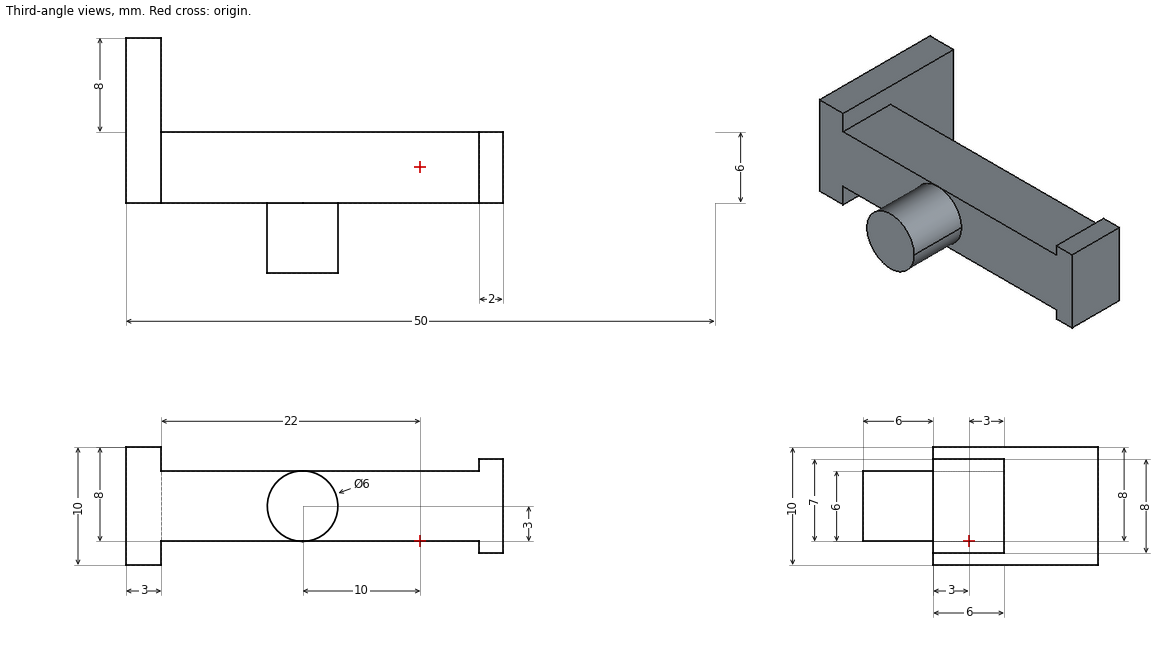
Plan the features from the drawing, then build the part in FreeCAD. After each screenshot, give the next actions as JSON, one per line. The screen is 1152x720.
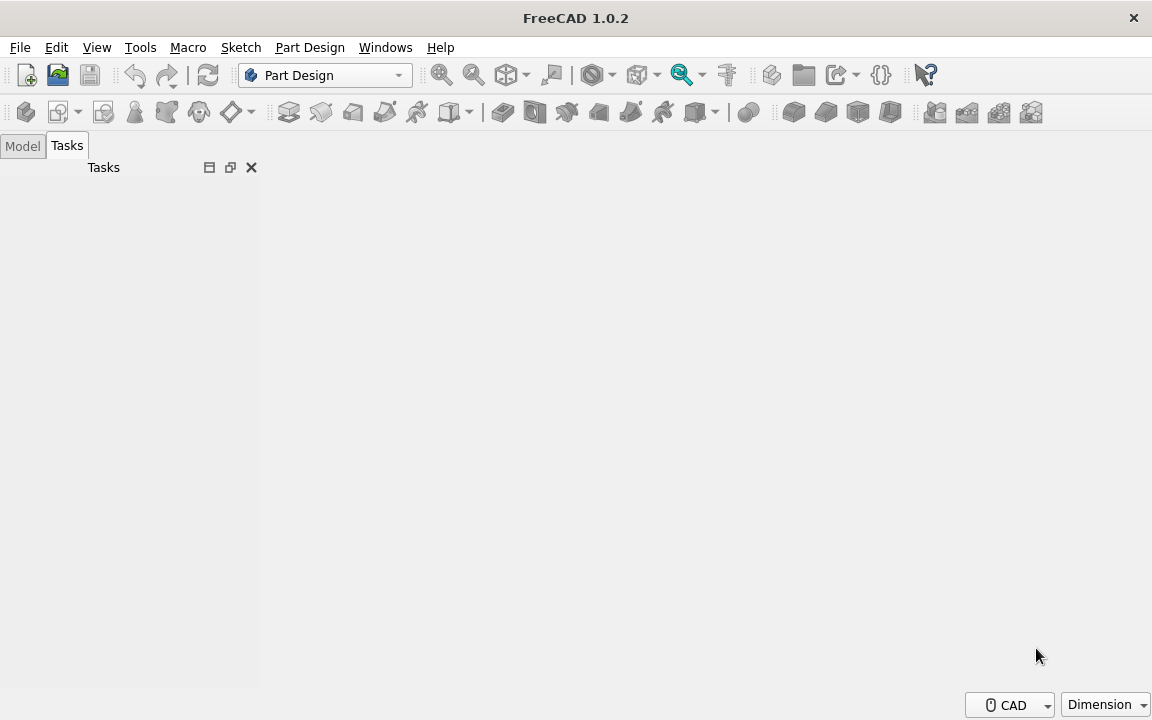
{"action": "left_click", "coordinate": [26, 76]}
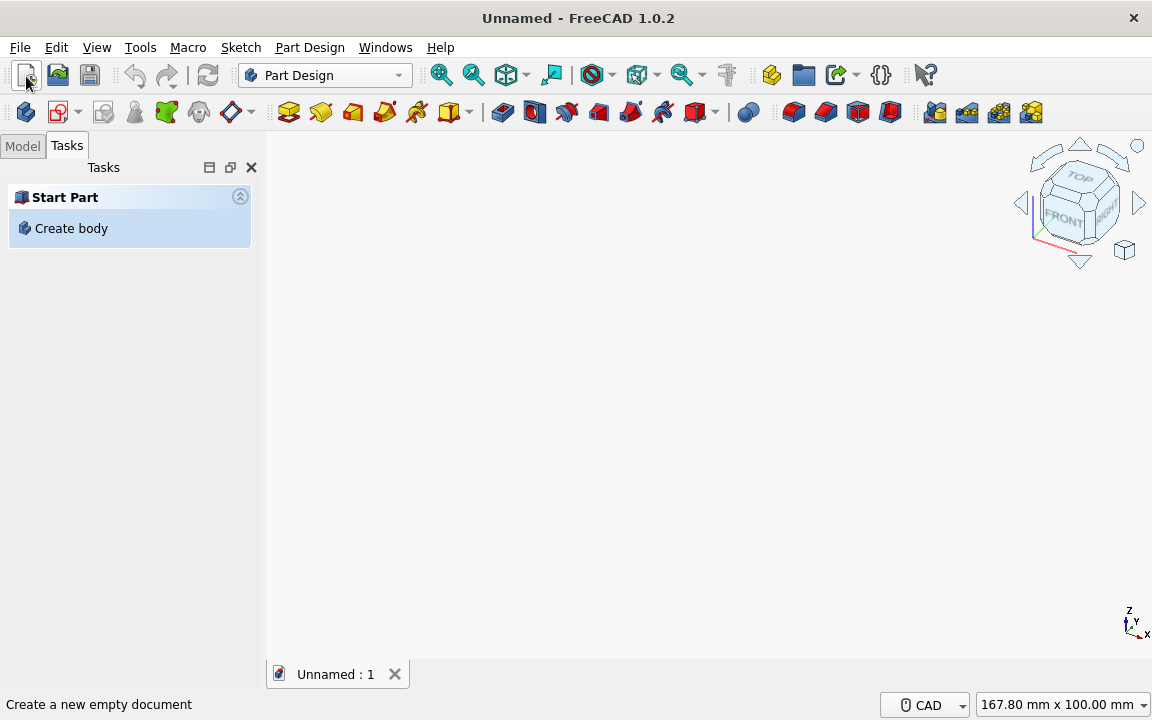
{"action": "left_click", "coordinate": [58, 112]}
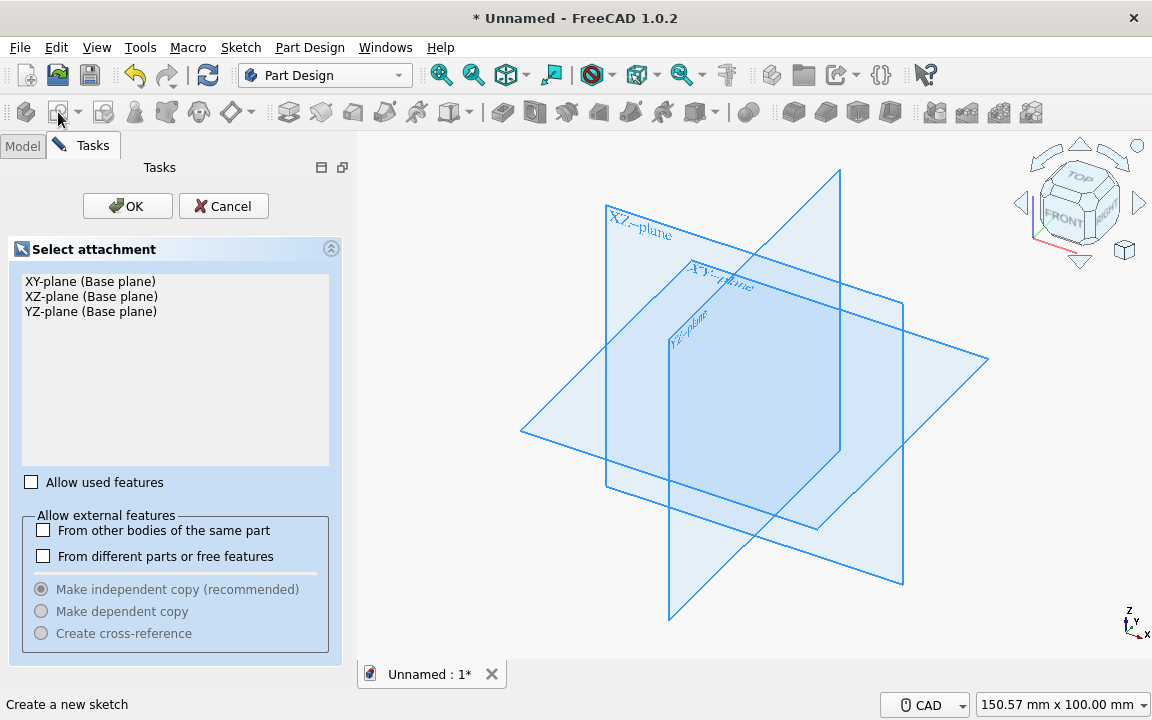
{"action": "left_click", "coordinate": [82, 282]}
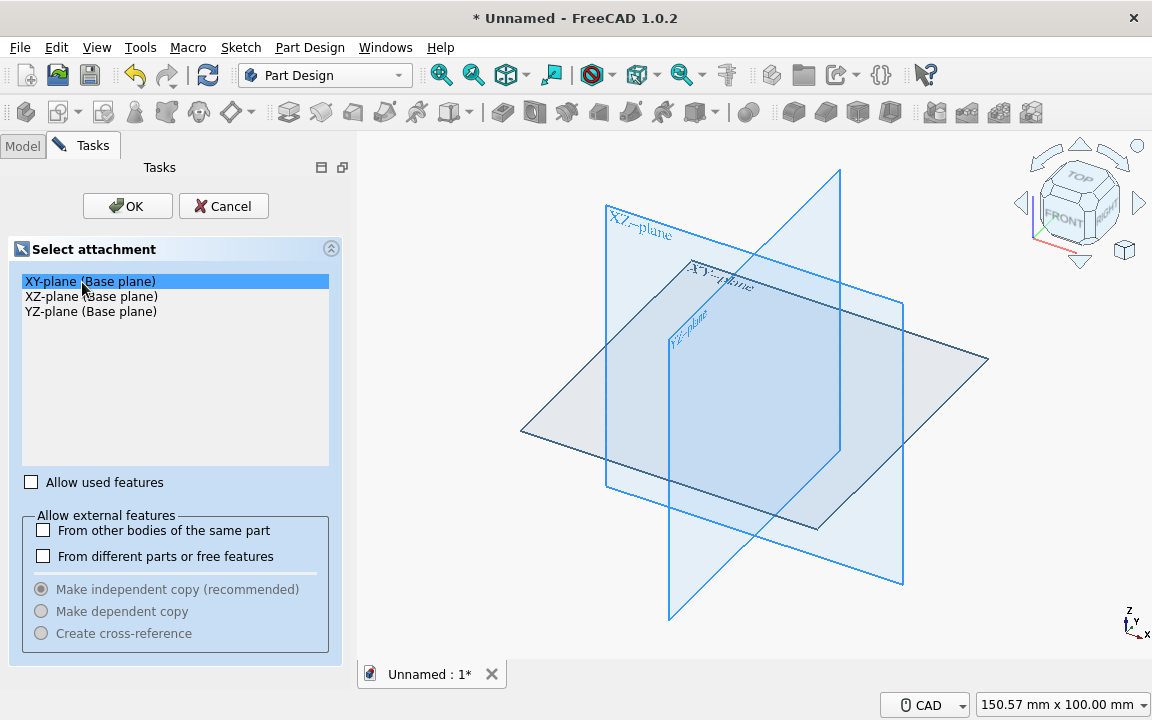
{"action": "left_click", "coordinate": [128, 206]}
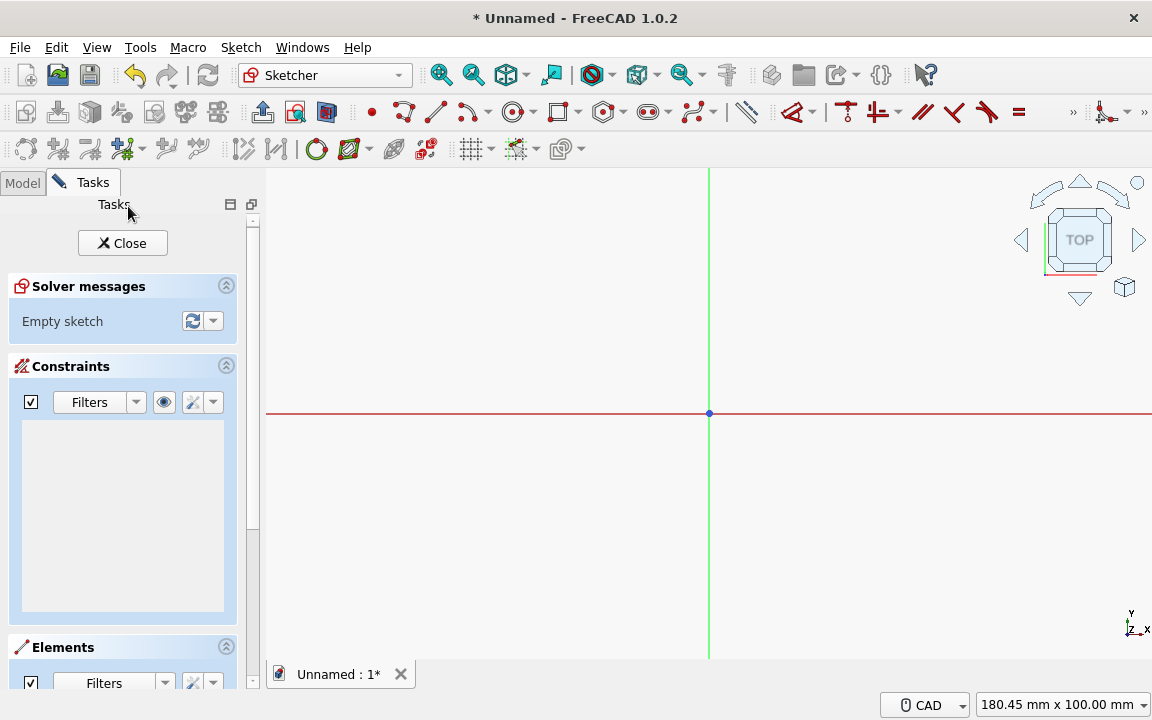
{"action": "scroll", "coordinate": [792, 414], "scroll_direction": "up", "scroll_amount": 3}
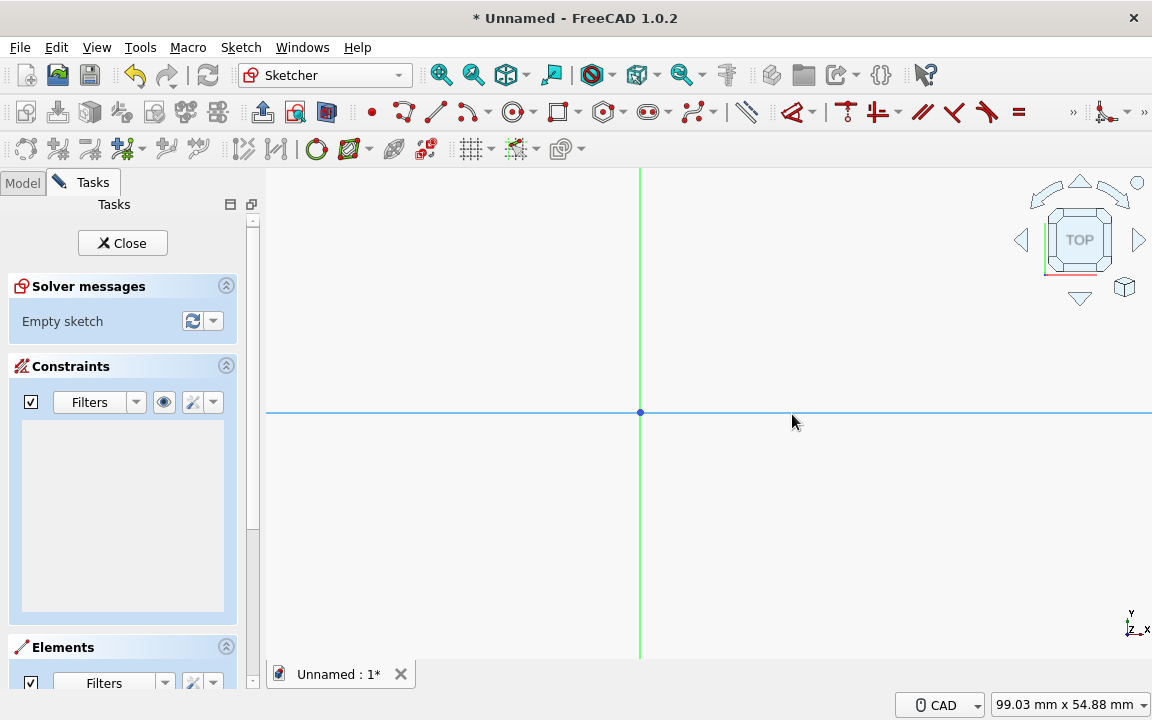
{"action": "key", "text": "g v"}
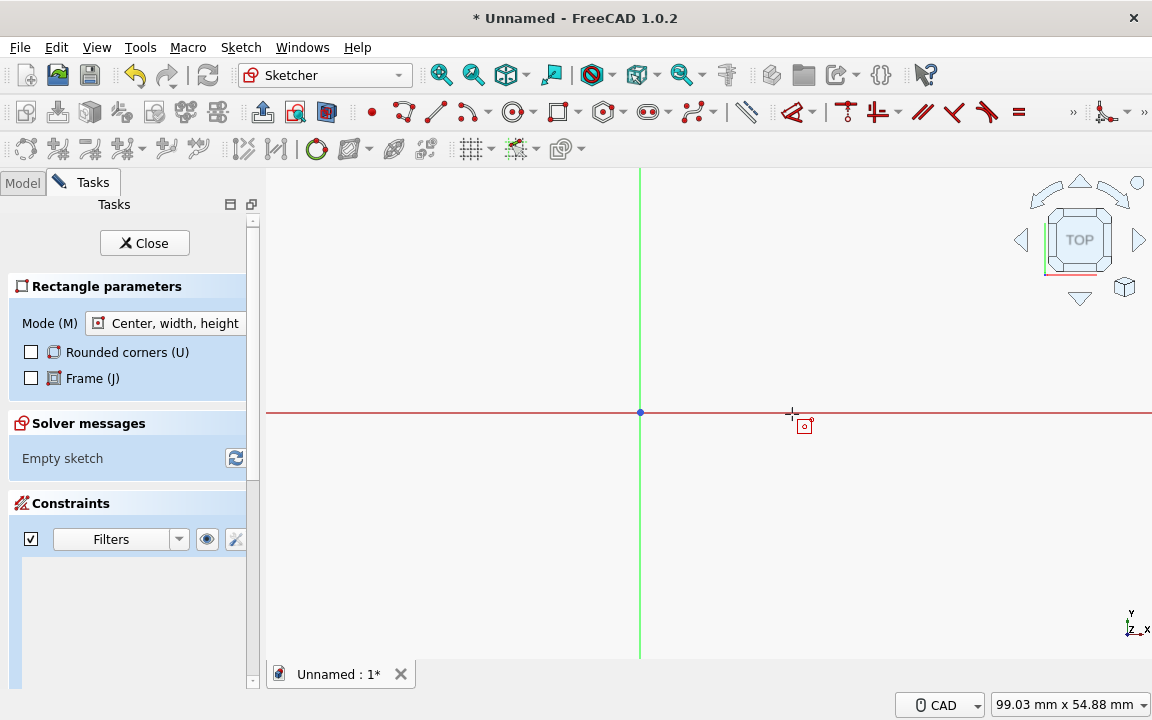
{"action": "left_click", "coordinate": [640, 413]}
{"action": "mouse_move", "coordinate": [864, 386]}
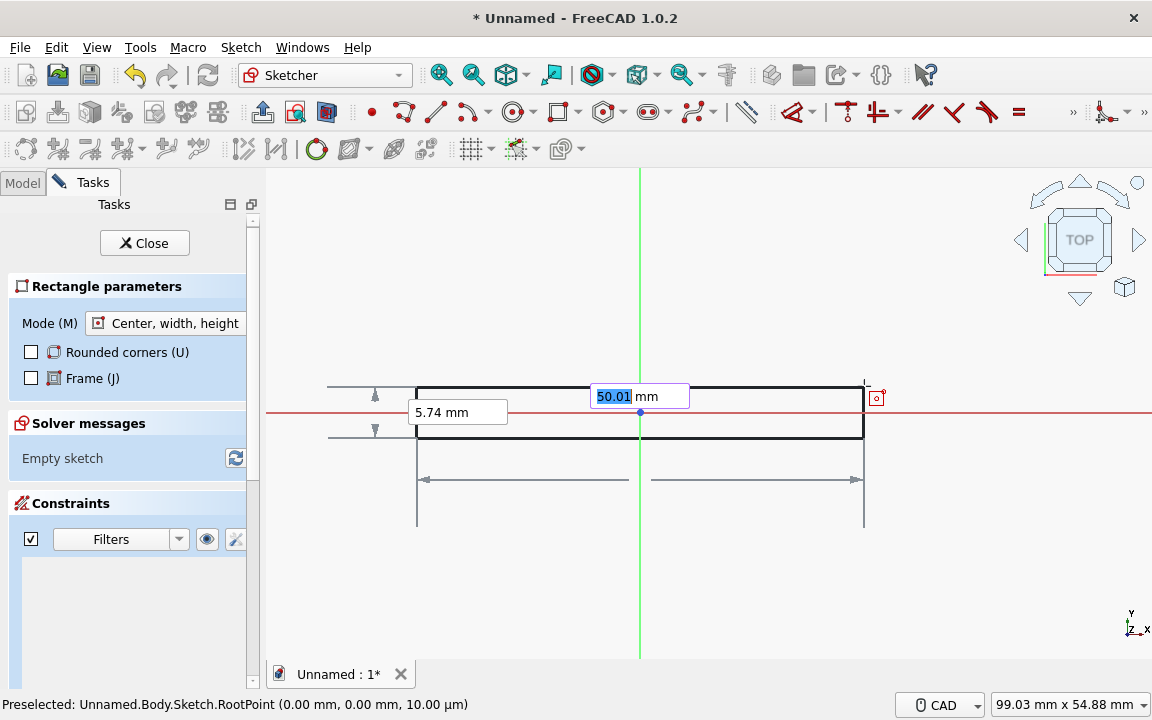
{"action": "type", "text": "50"}
{"action": "key", "text": "Tab"}
{"action": "type", "text": "6"}
{"action": "key", "text": "Return"}
{"action": "key", "text": "Escape"}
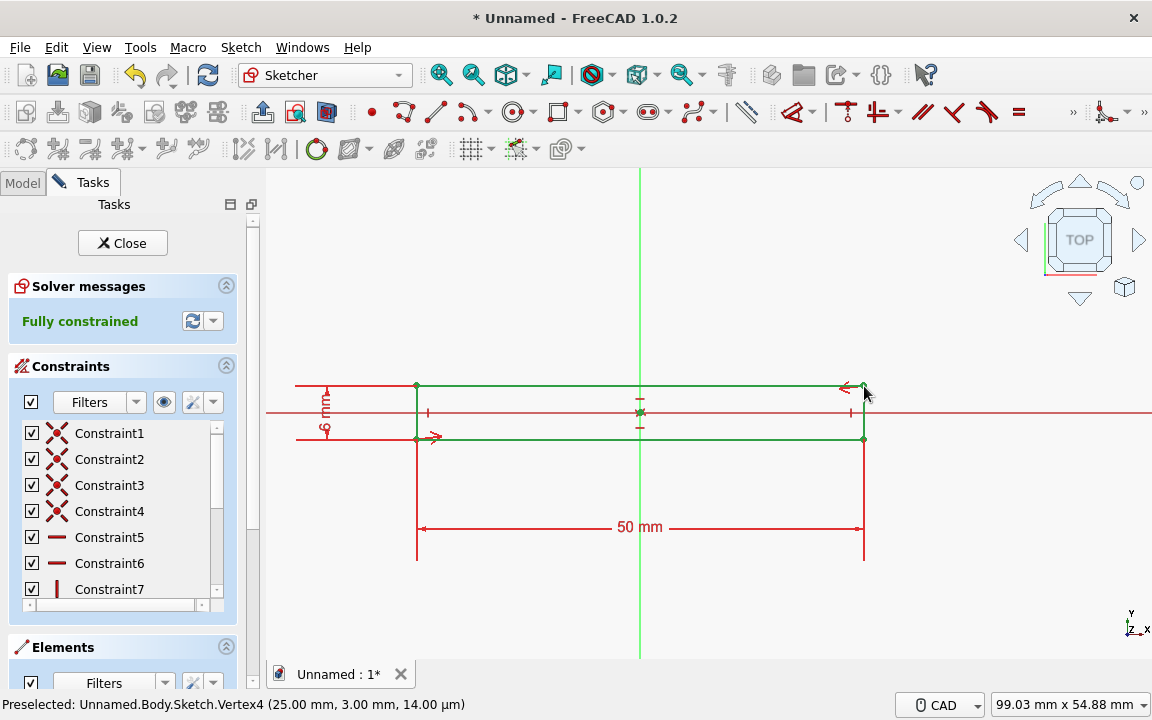
{"action": "left_click", "coordinate": [123, 243]}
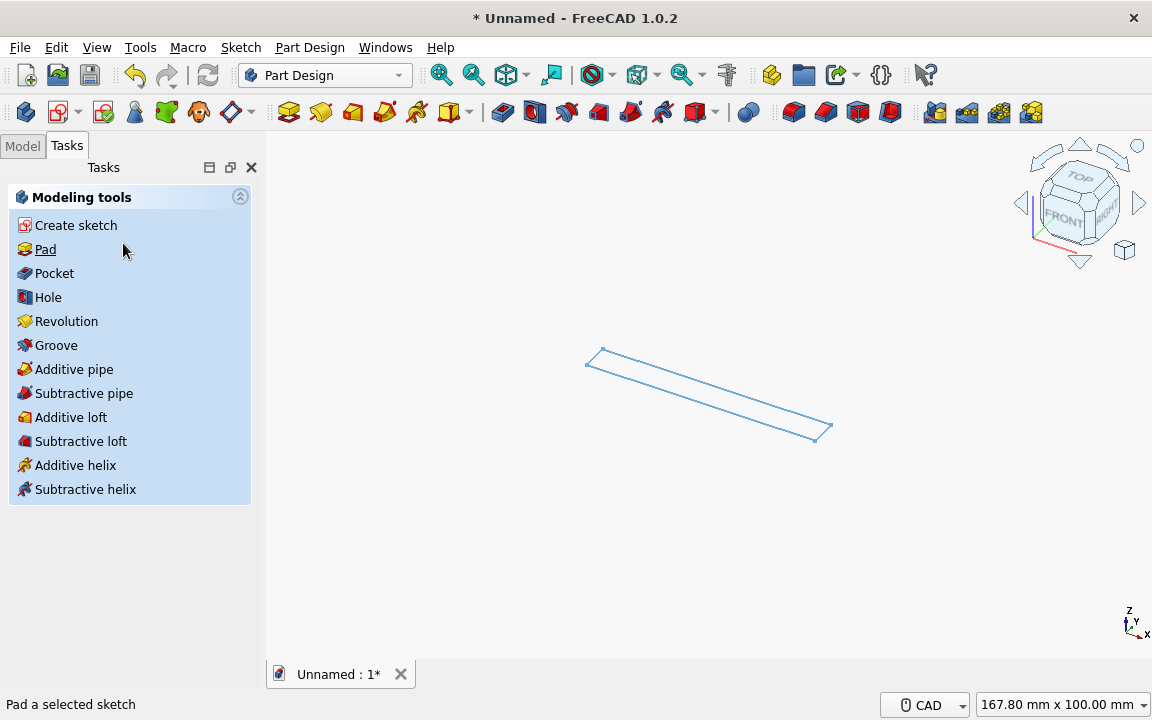
{"action": "left_click", "coordinate": [290, 112]}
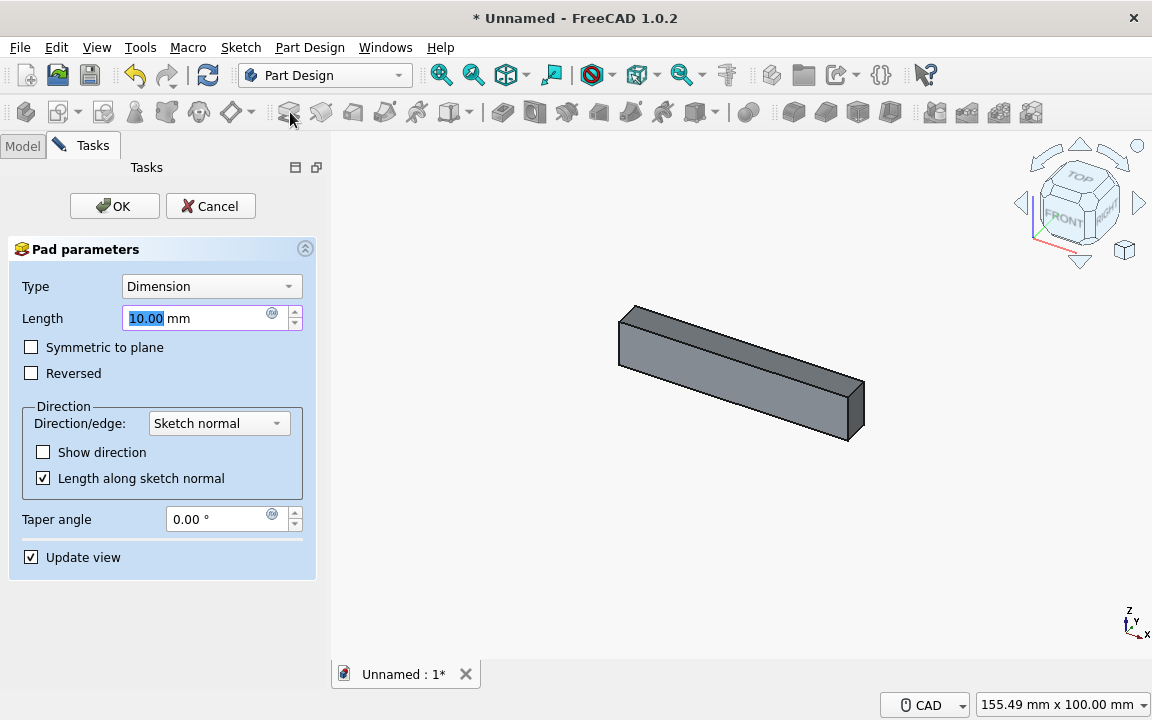
{"action": "type", "text": "6"}
{"action": "key", "text": "Tab"}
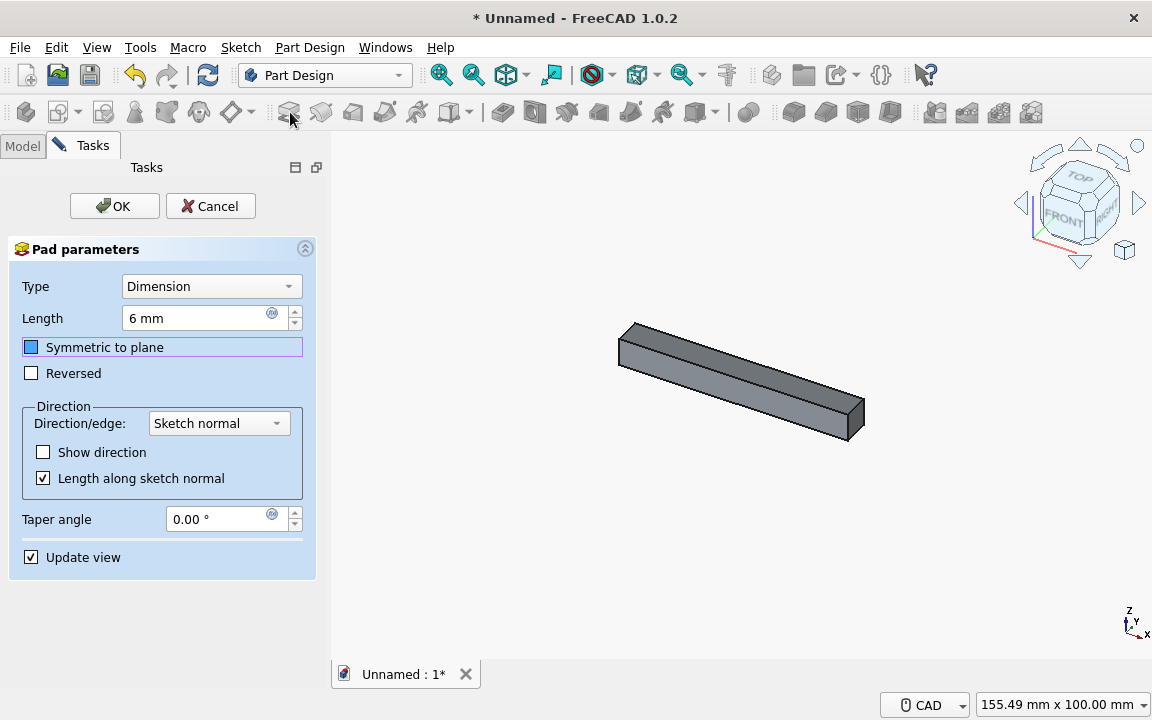
{"action": "left_click", "coordinate": [115, 206]}